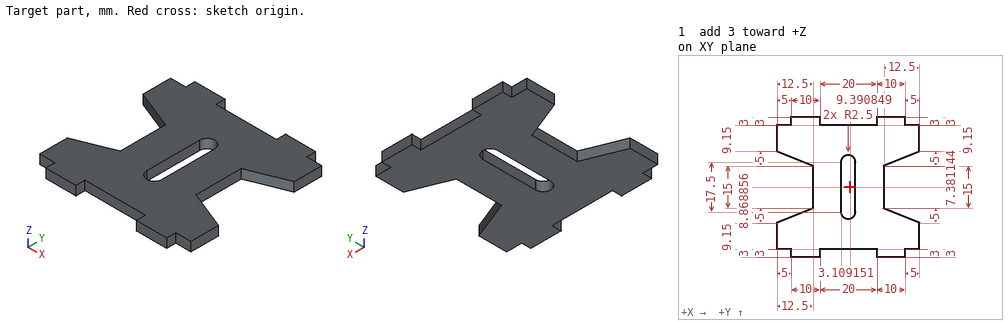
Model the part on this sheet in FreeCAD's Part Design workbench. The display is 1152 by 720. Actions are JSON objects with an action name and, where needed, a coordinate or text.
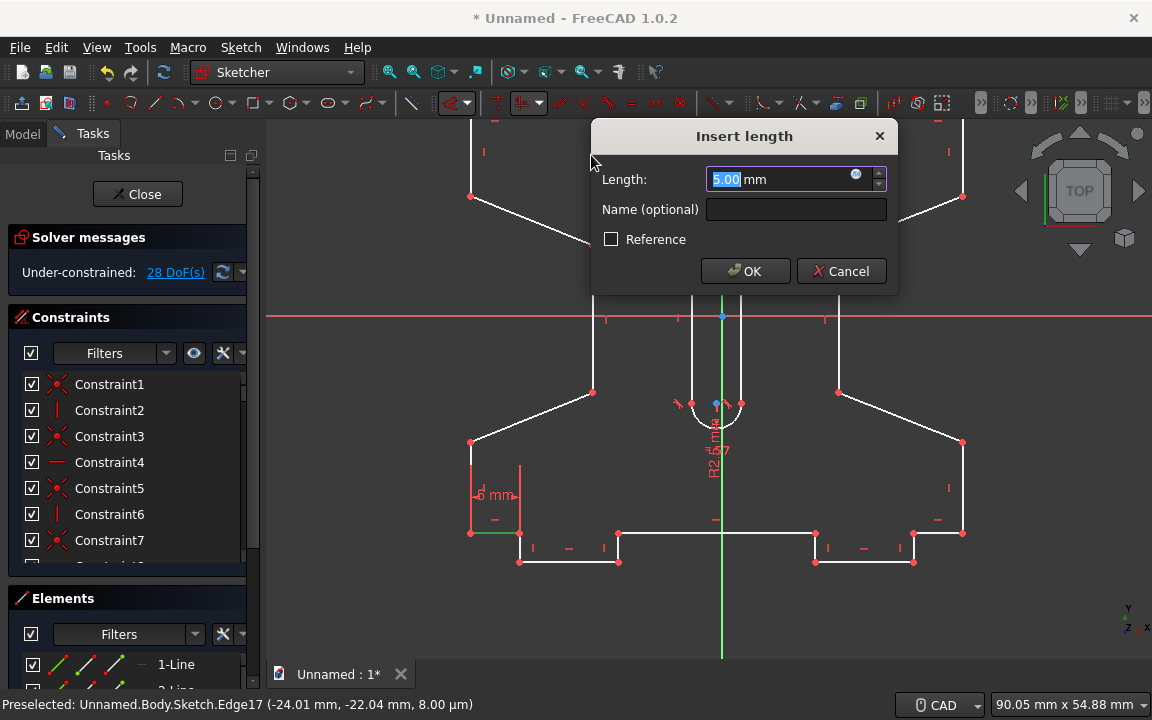
{"action": "type", "text": "5"}
{"action": "key", "text": "Return"}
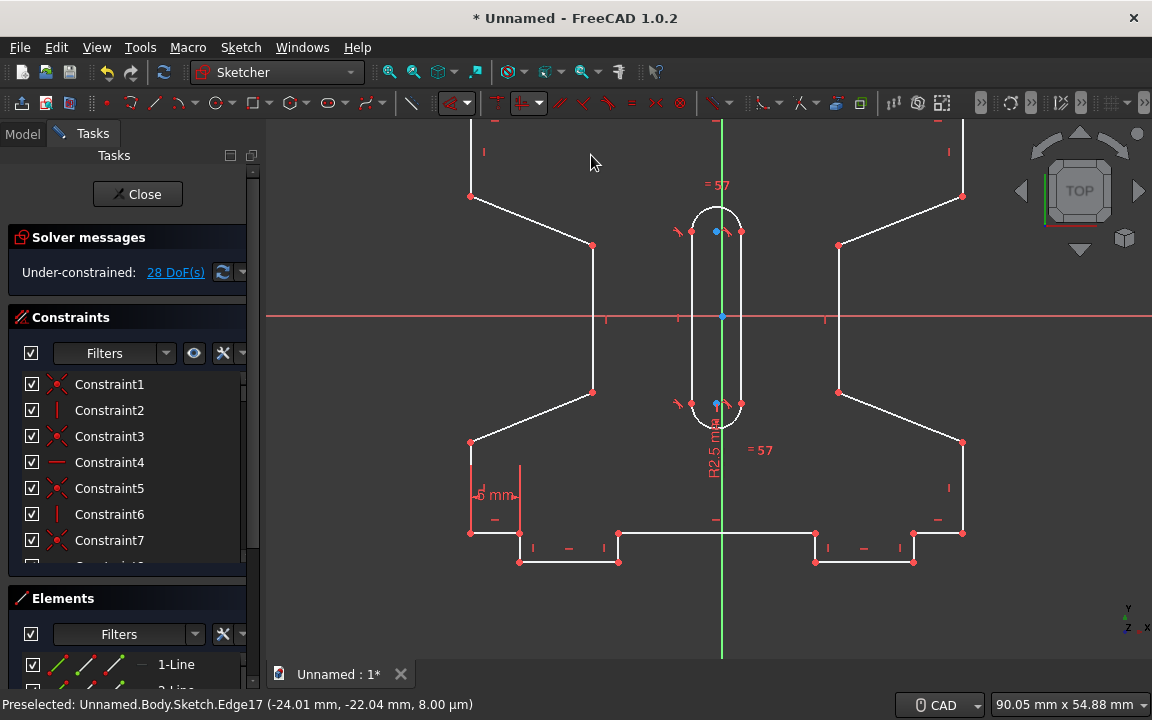
{"action": "scroll", "coordinate": [520, 545], "scroll_direction": "up", "scroll_amount": 2}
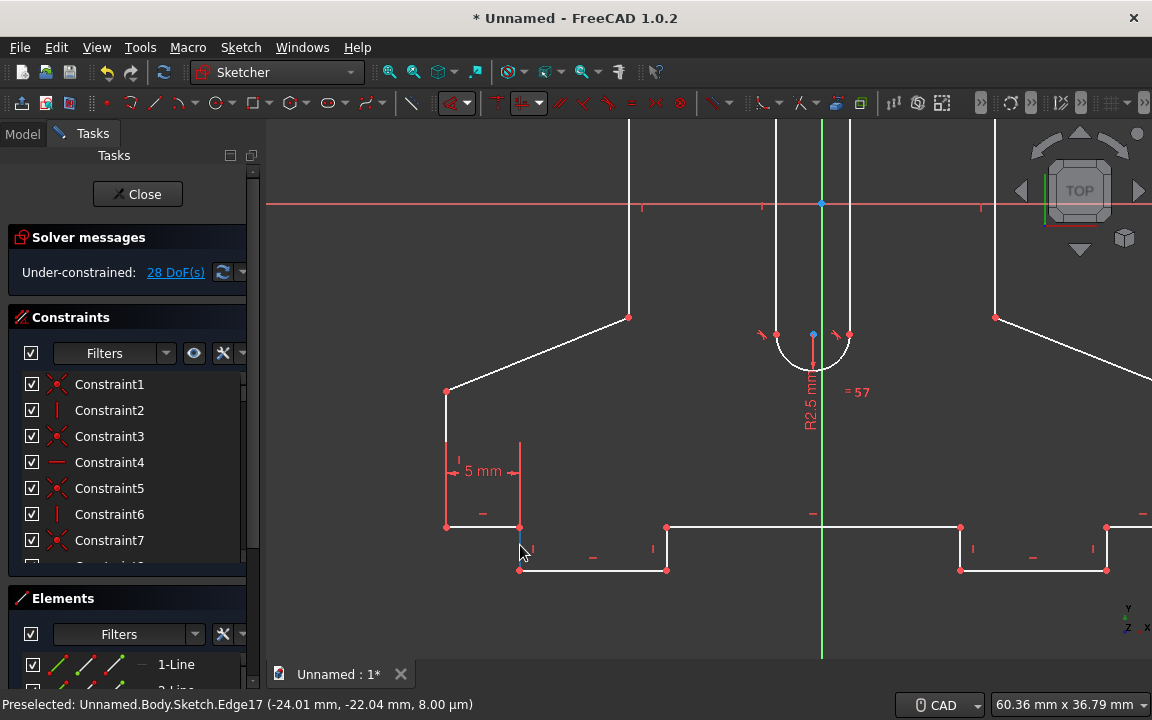
{"action": "left_click", "coordinate": [520, 544]}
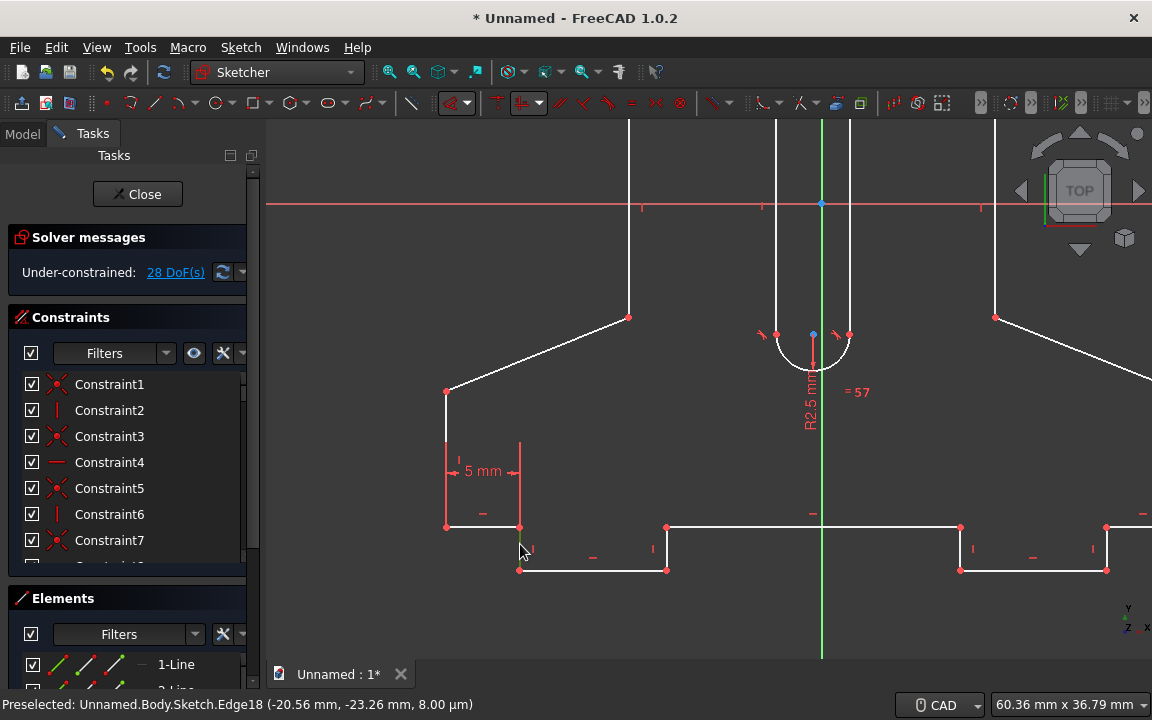
{"action": "left_click", "coordinate": [470, 104]}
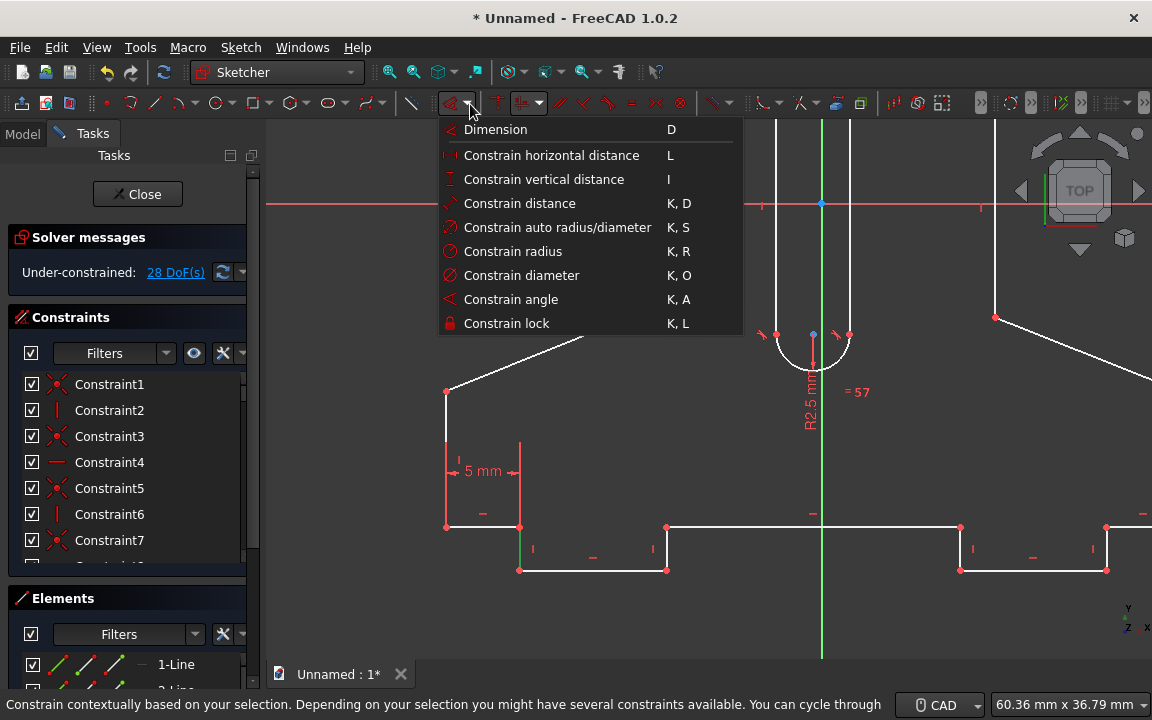
{"action": "left_click", "coordinate": [591, 179]}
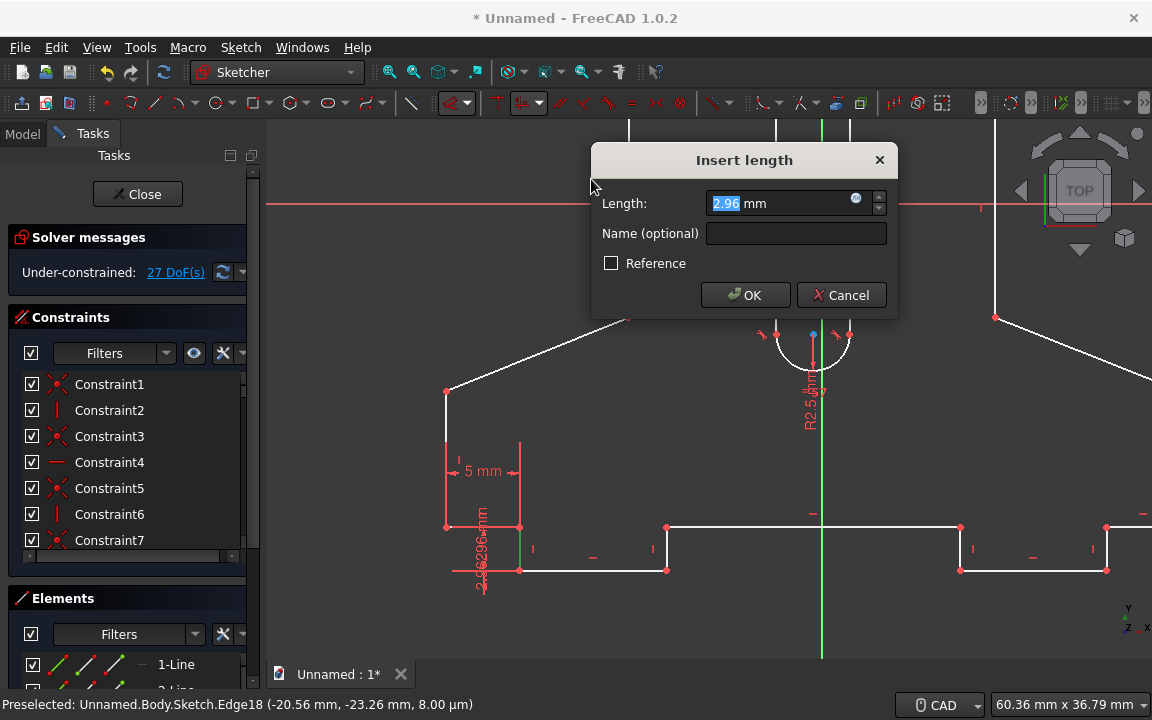
{"action": "type", "text": "3"}
{"action": "key", "text": "Return"}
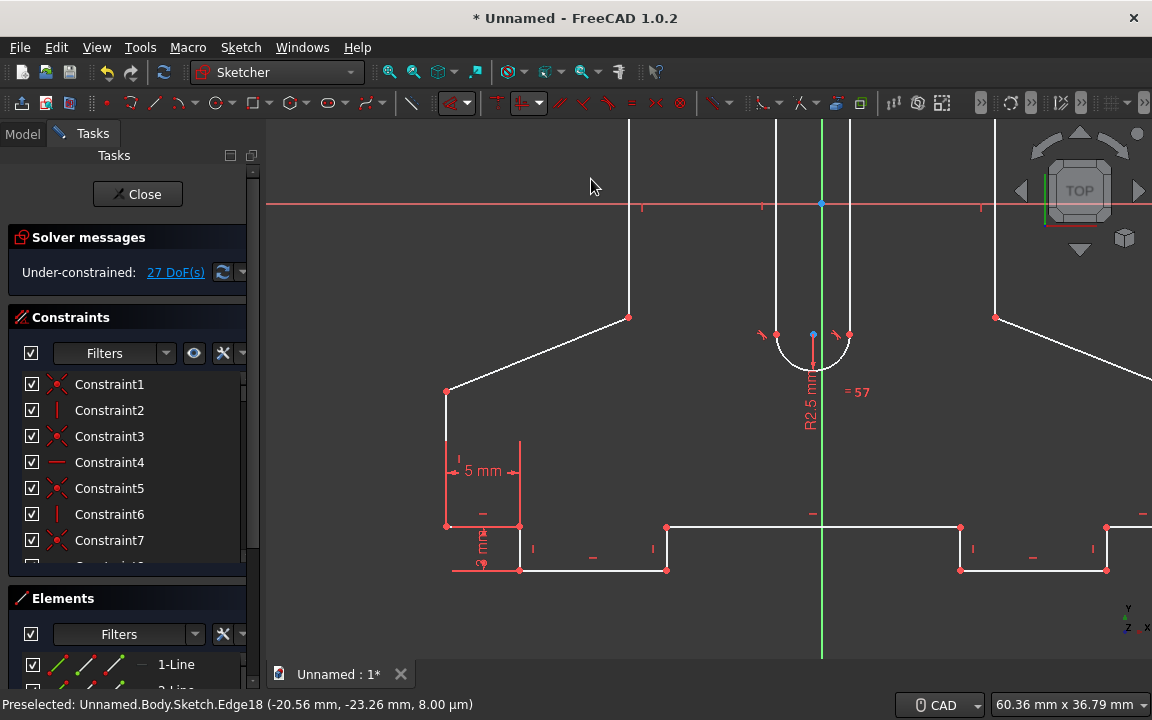
{"action": "left_click", "coordinate": [667, 557]}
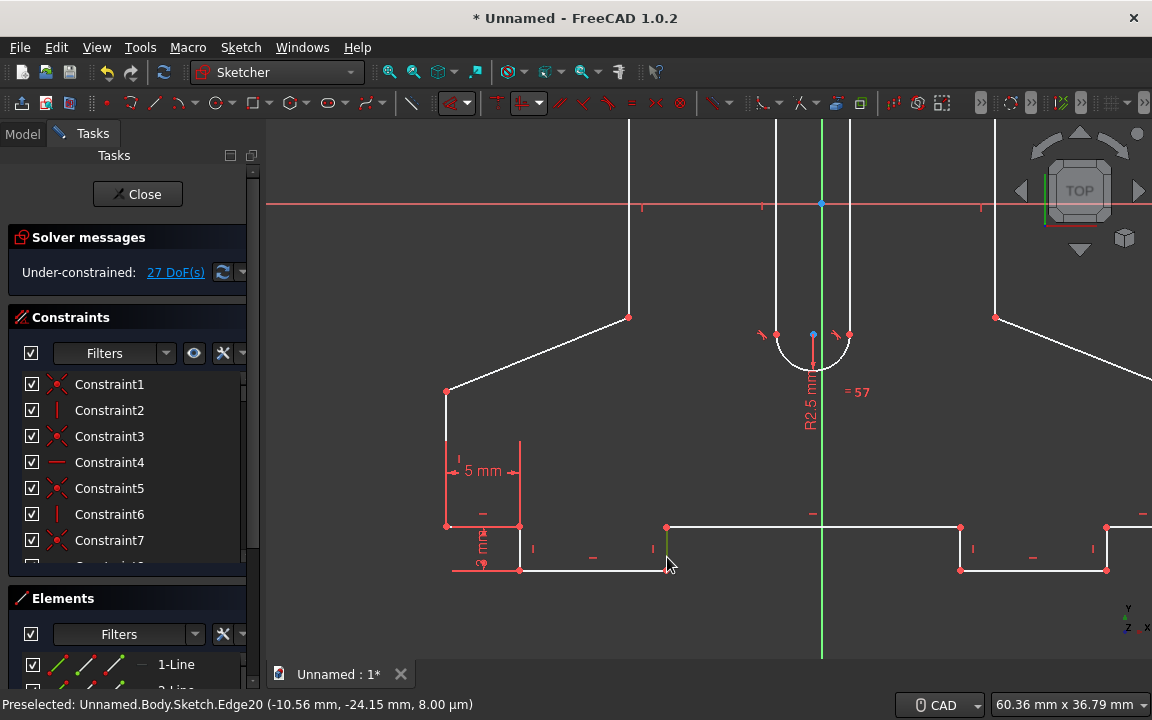
{"action": "key", "text": "i"}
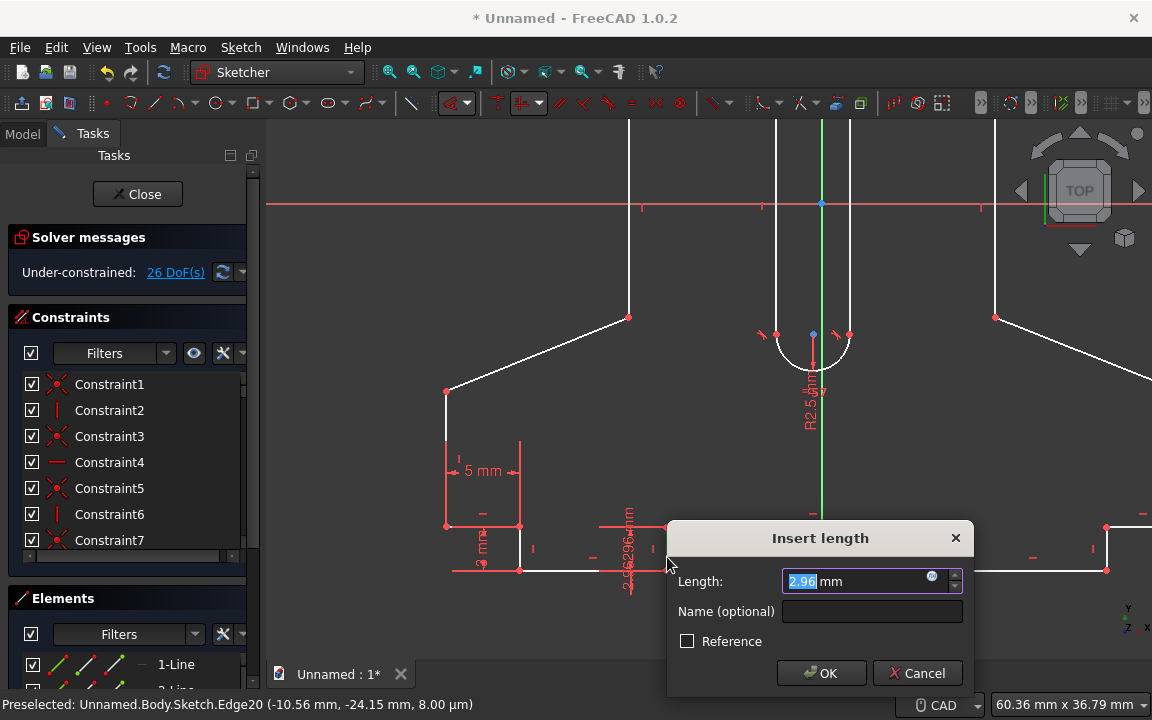
{"action": "type", "text": "3"}
{"action": "key", "text": "Return"}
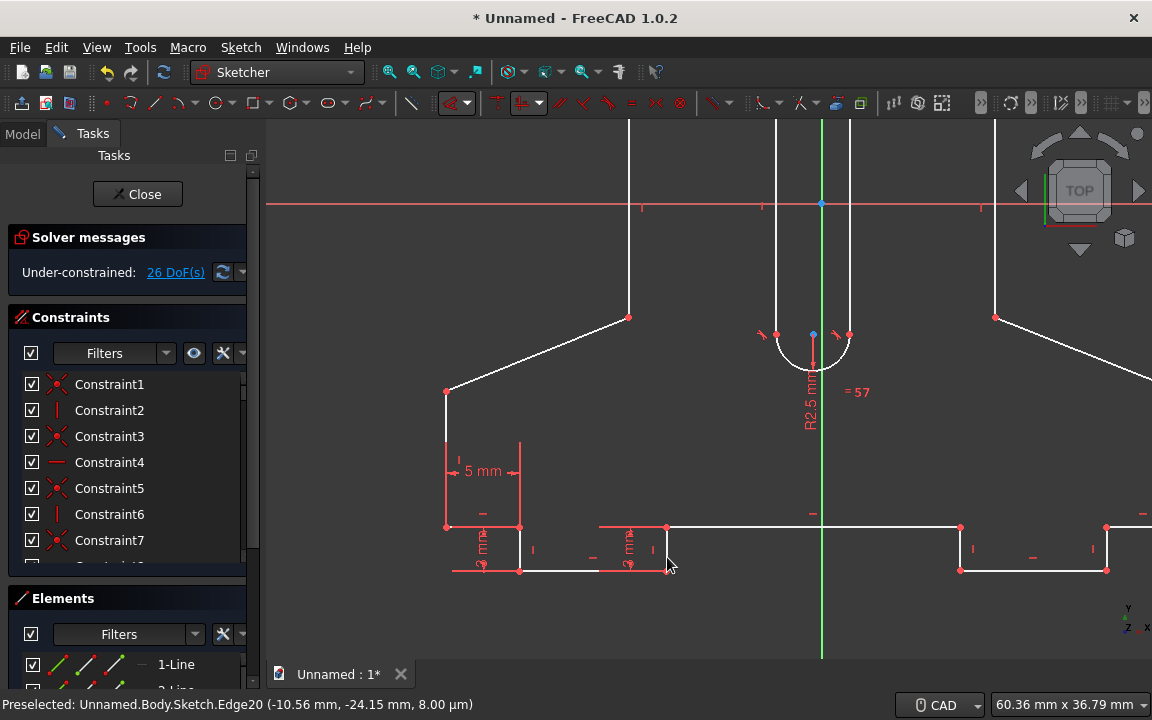
{"action": "left_click", "coordinate": [960, 540]}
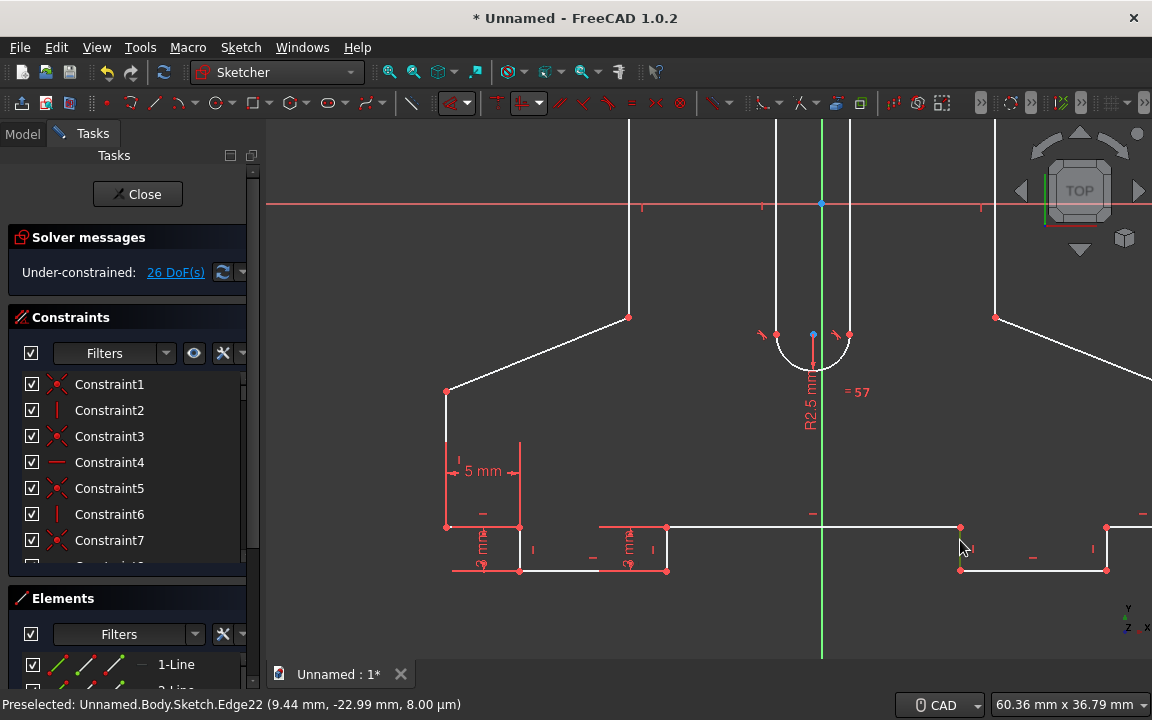
{"action": "key", "text": "i"}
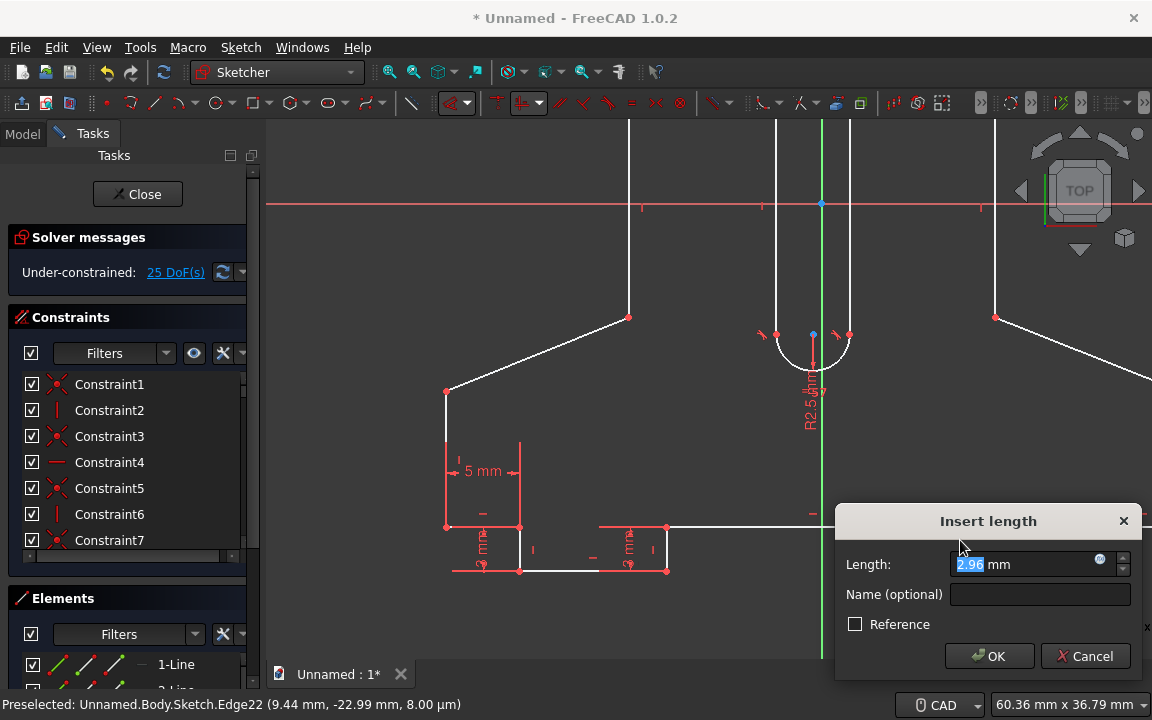
{"action": "type", "text": "3"}
{"action": "key", "text": "Return"}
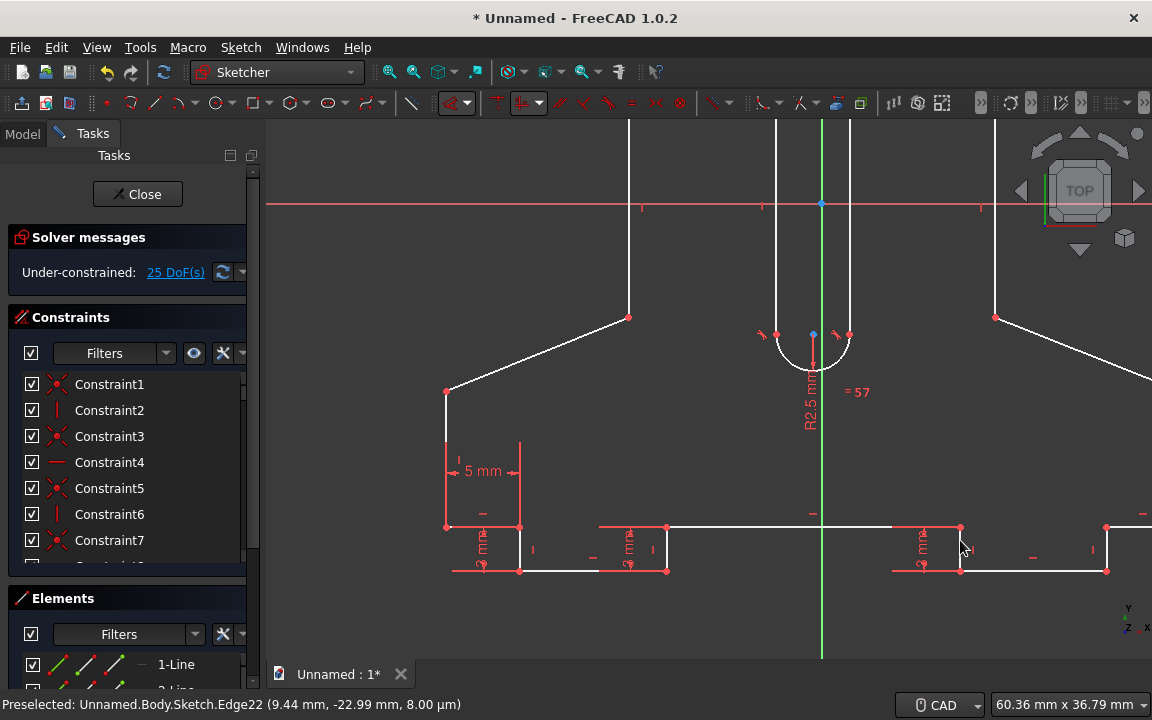
{"action": "scroll", "coordinate": [500, 539], "scroll_direction": "down", "scroll_amount": 4}